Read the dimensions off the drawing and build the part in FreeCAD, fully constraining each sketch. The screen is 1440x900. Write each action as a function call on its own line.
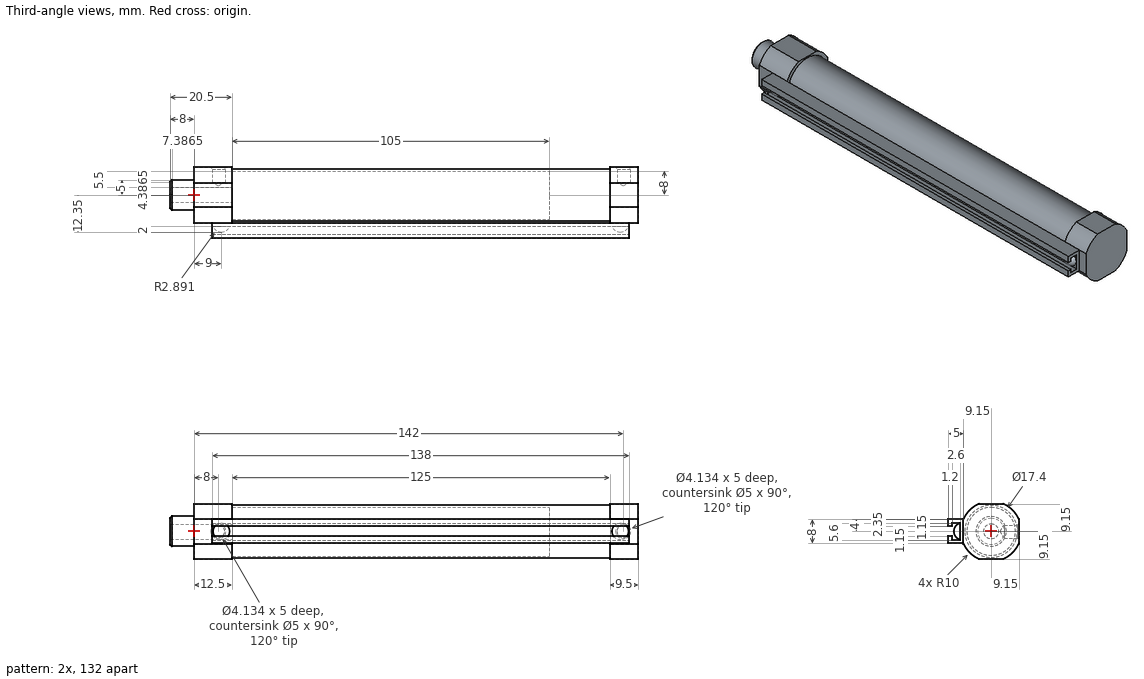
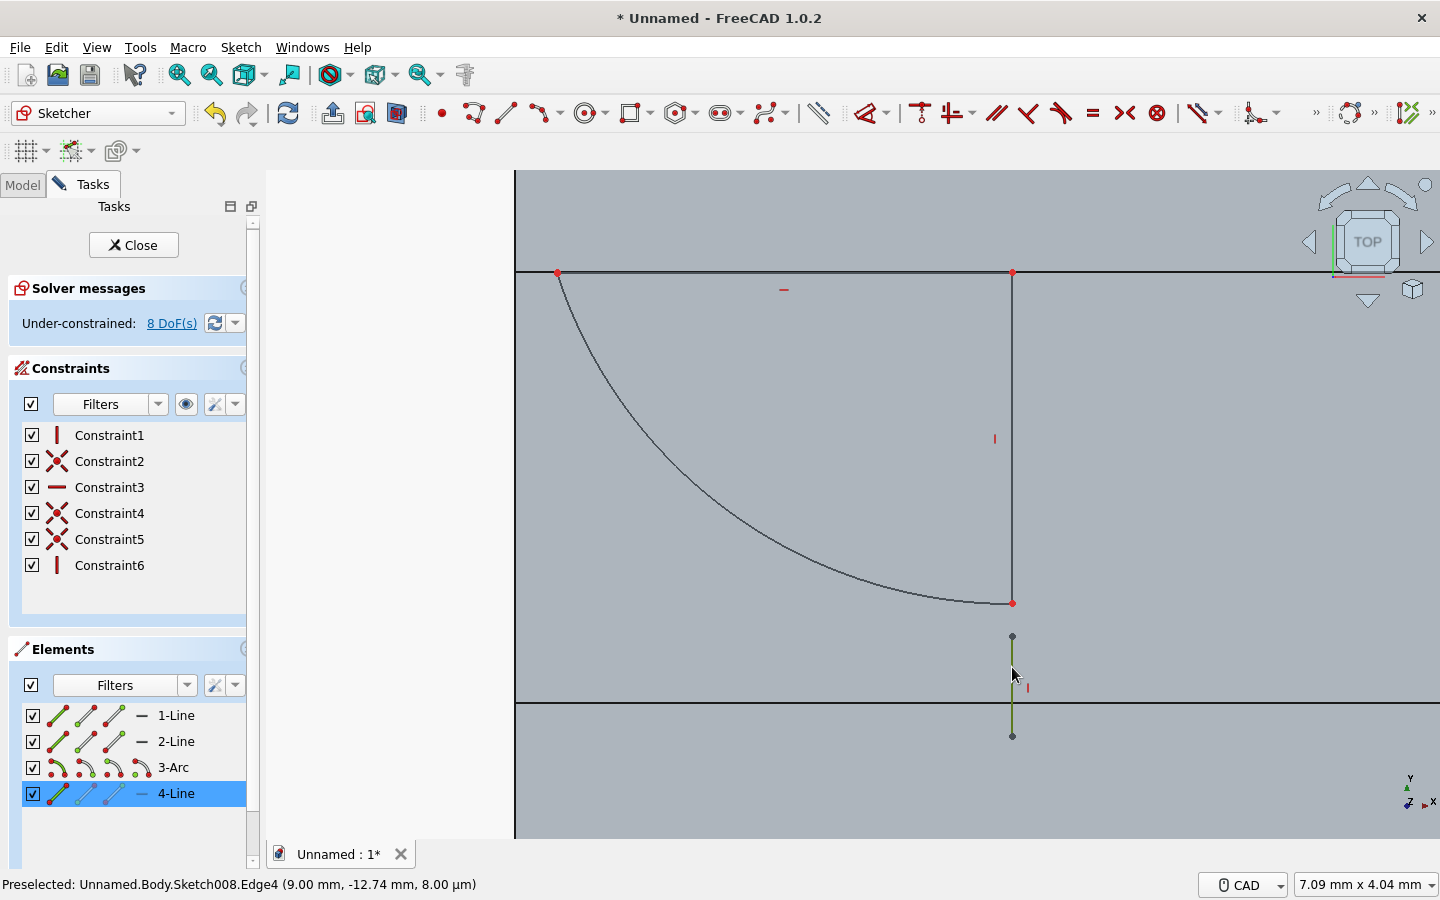
click(820, 114)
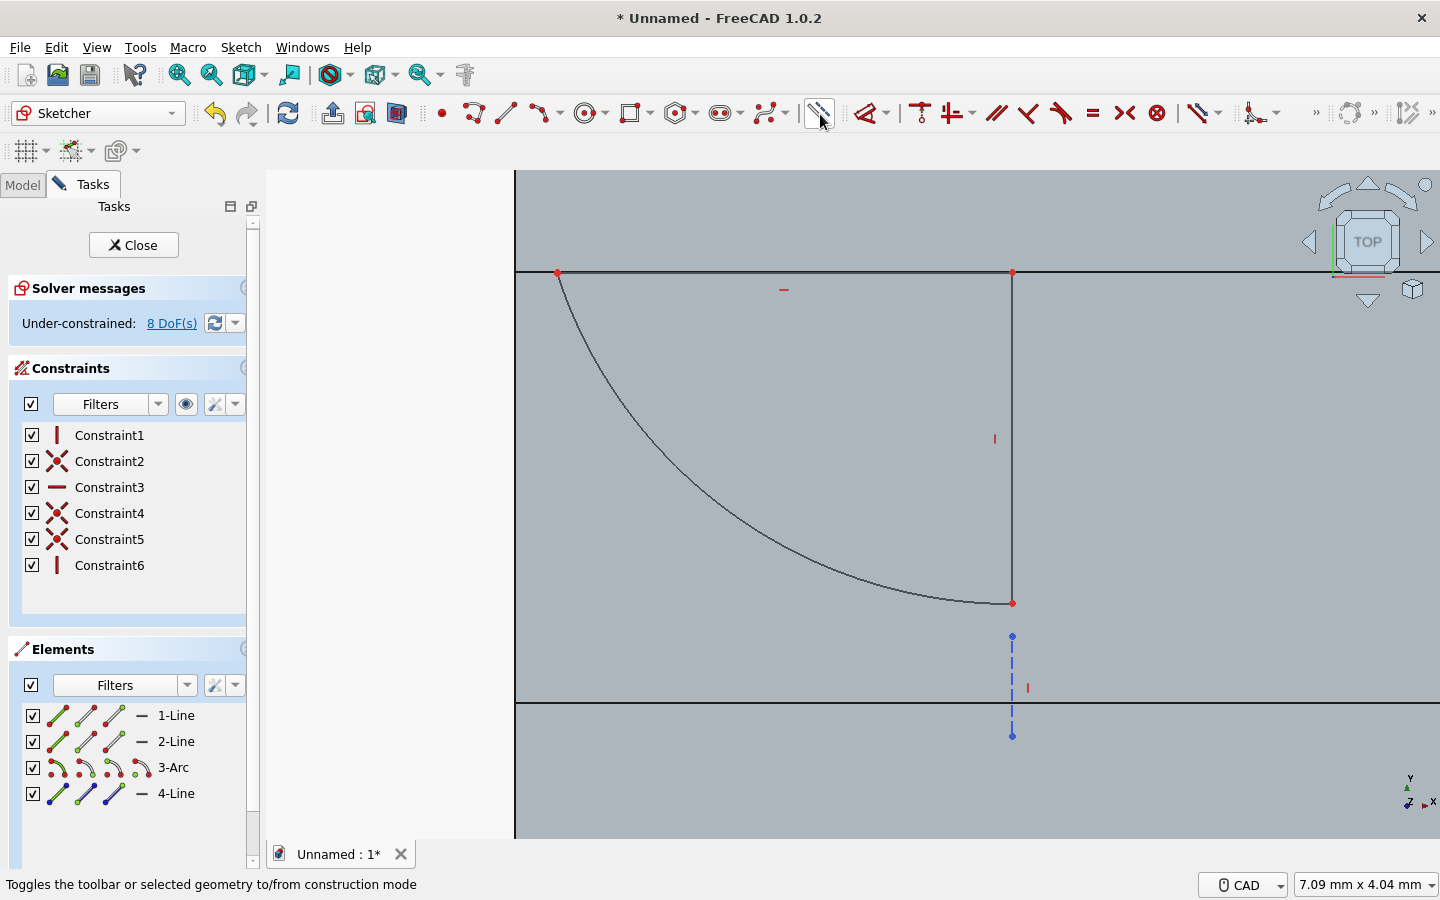
click(866, 114)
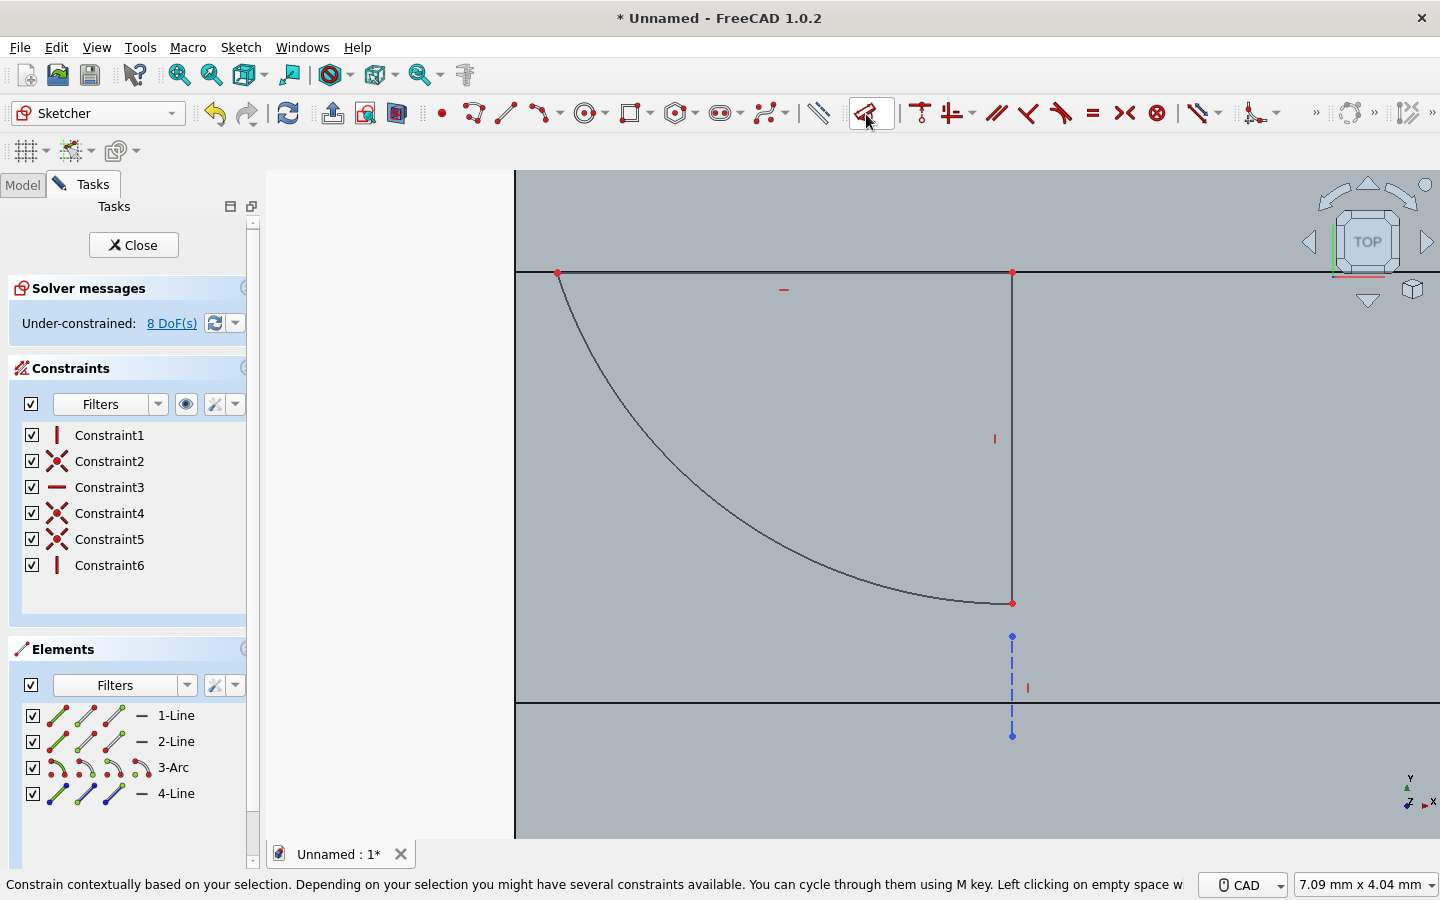
click(643, 430)
click(618, 450)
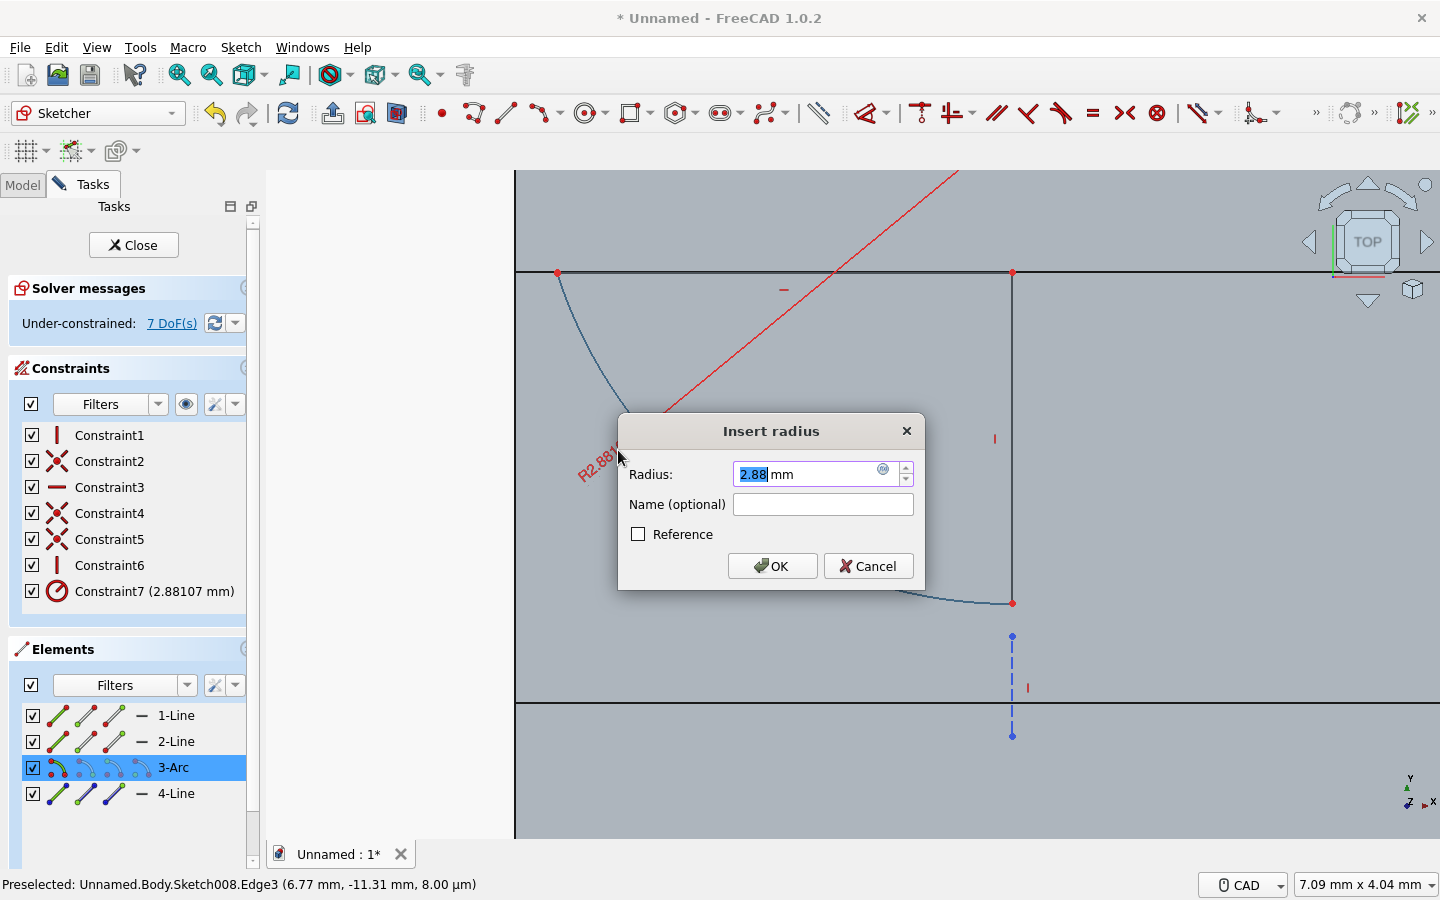
text(2.891)
key(Return)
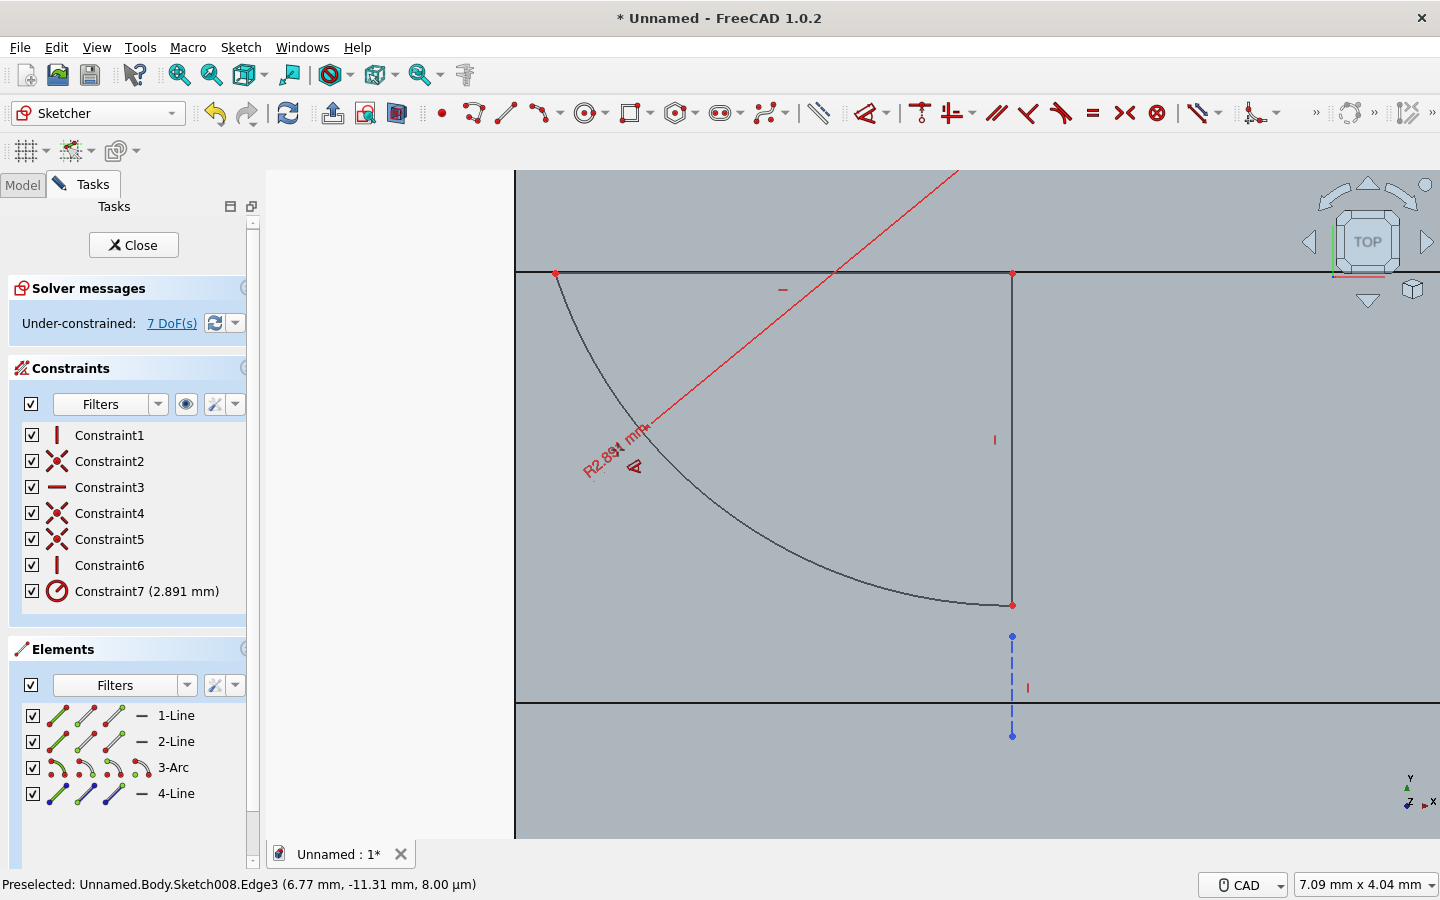
click(1012, 506)
click(1046, 439)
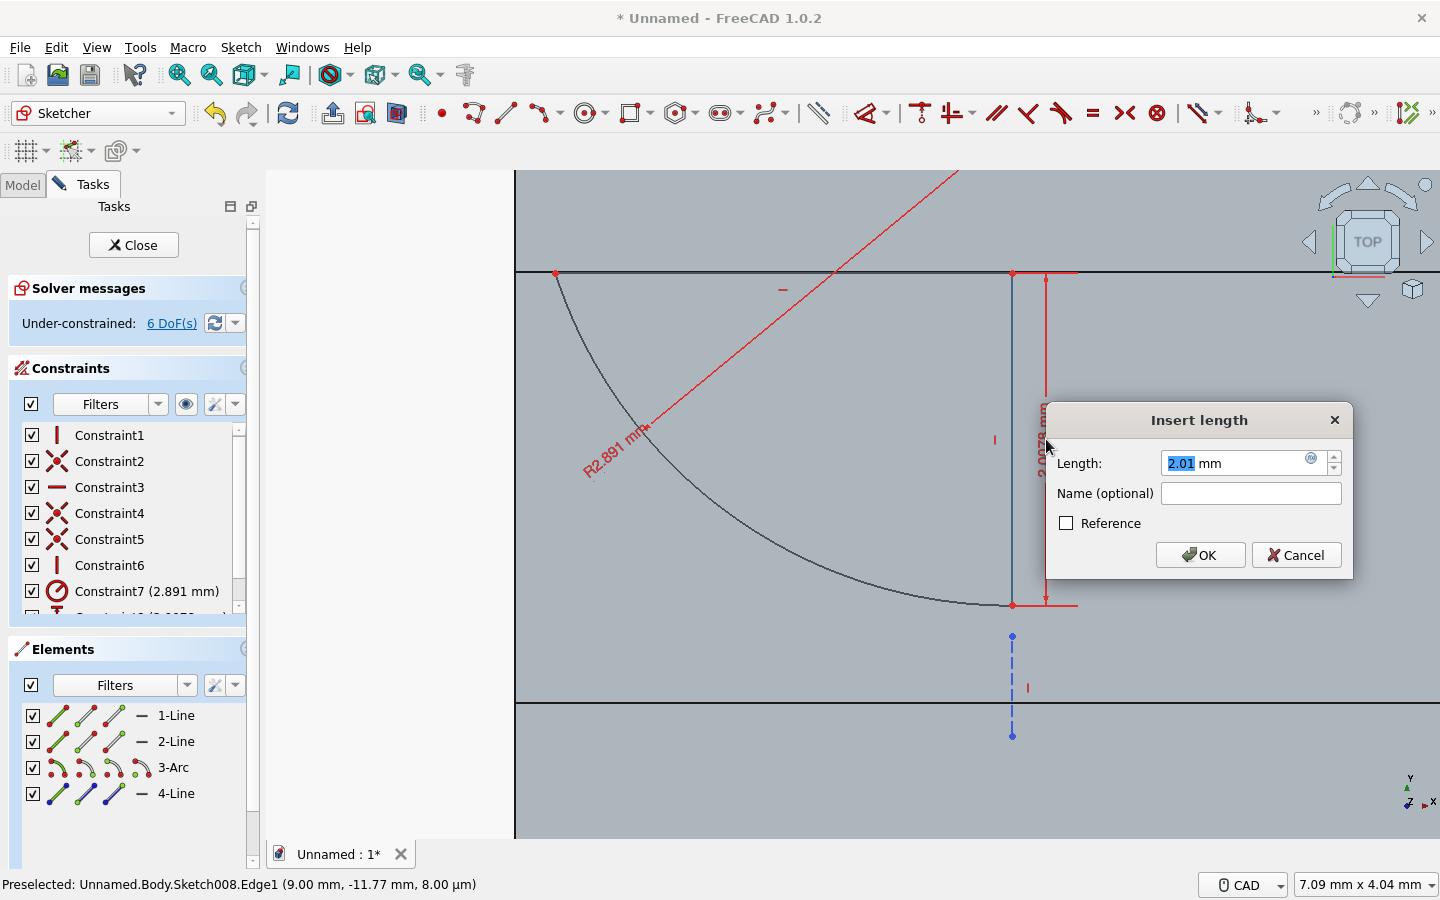
text(2)
key(Return)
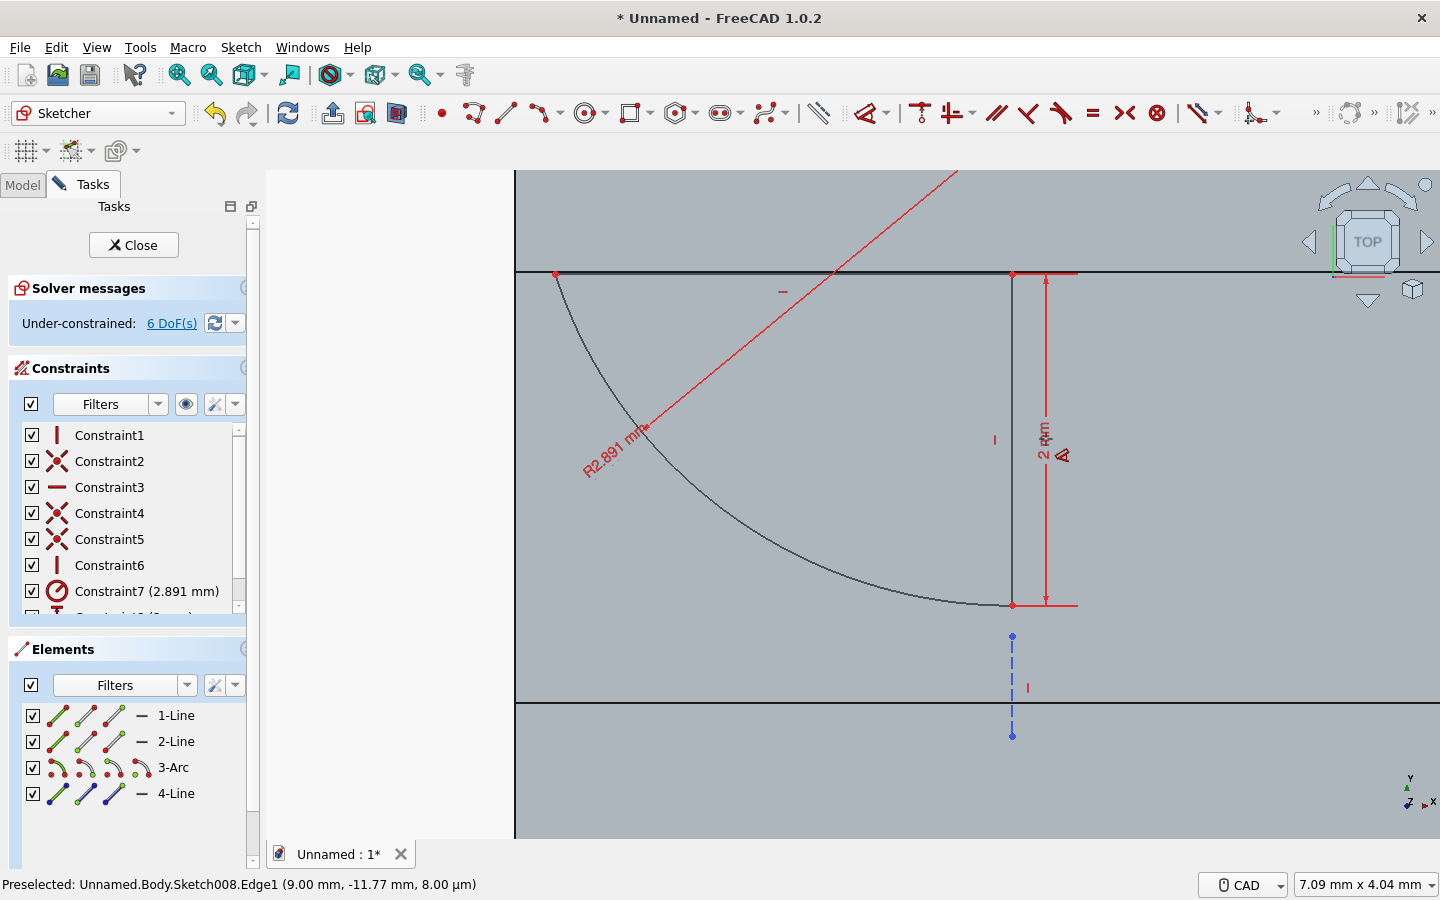
click(1012, 606)
click(653, 640)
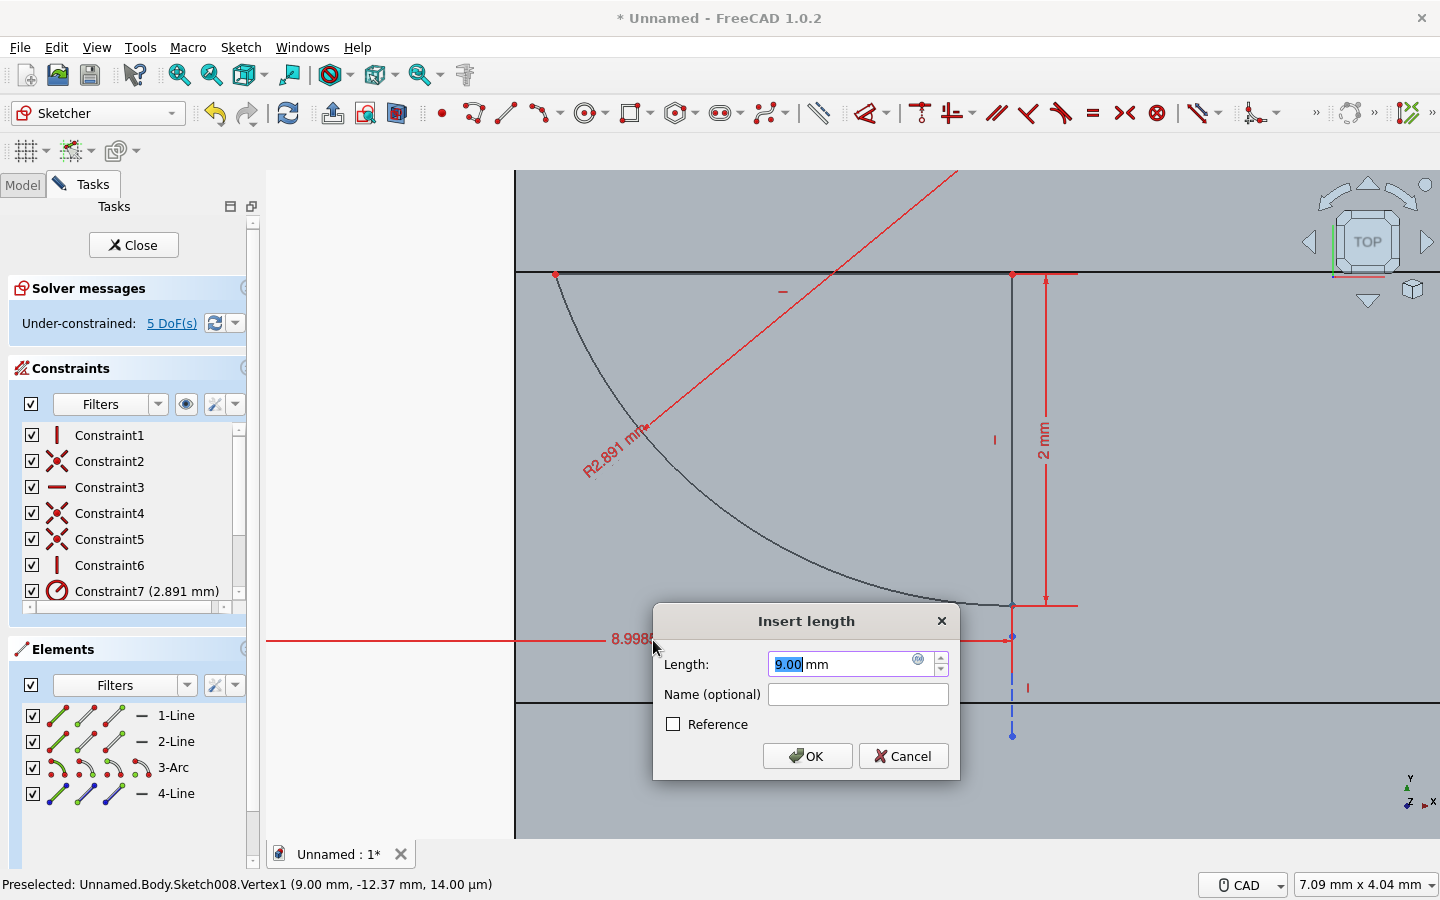
text(9)
key(Return)